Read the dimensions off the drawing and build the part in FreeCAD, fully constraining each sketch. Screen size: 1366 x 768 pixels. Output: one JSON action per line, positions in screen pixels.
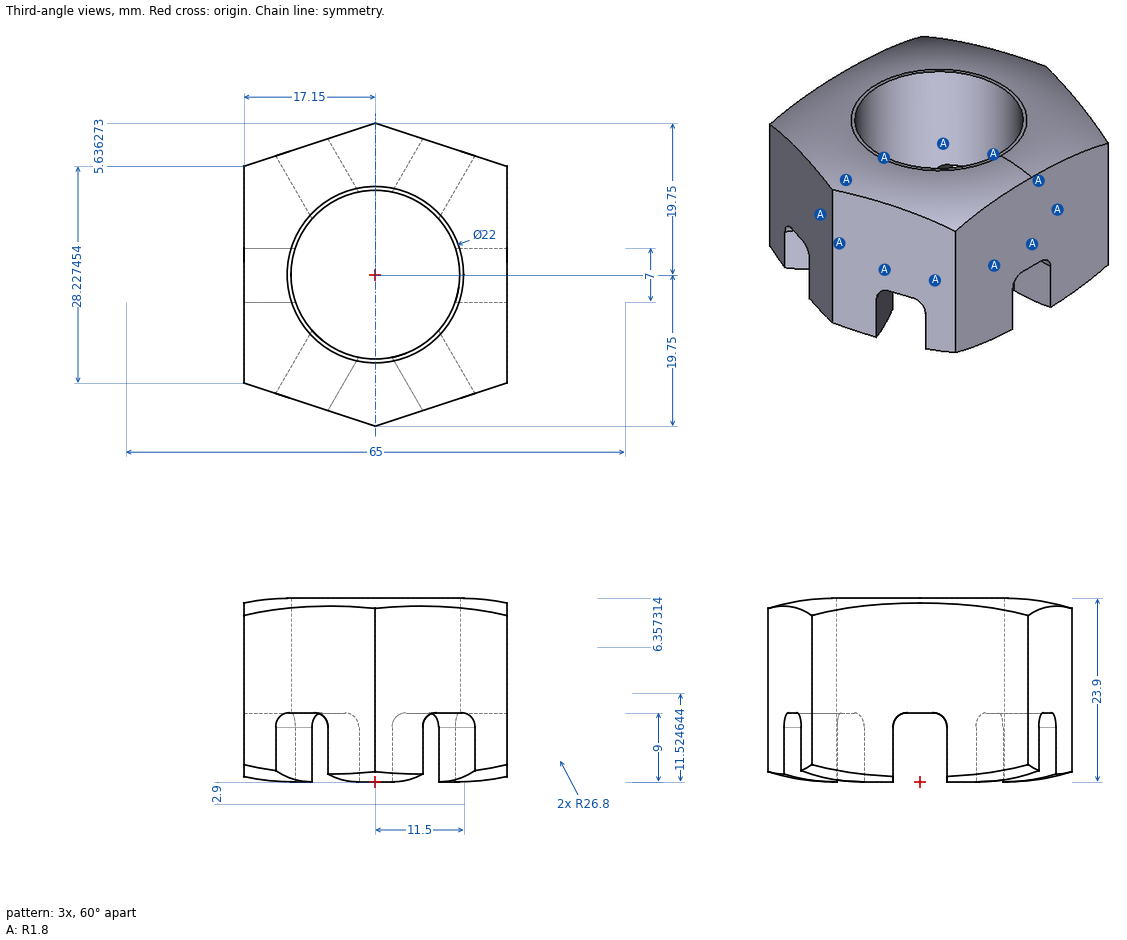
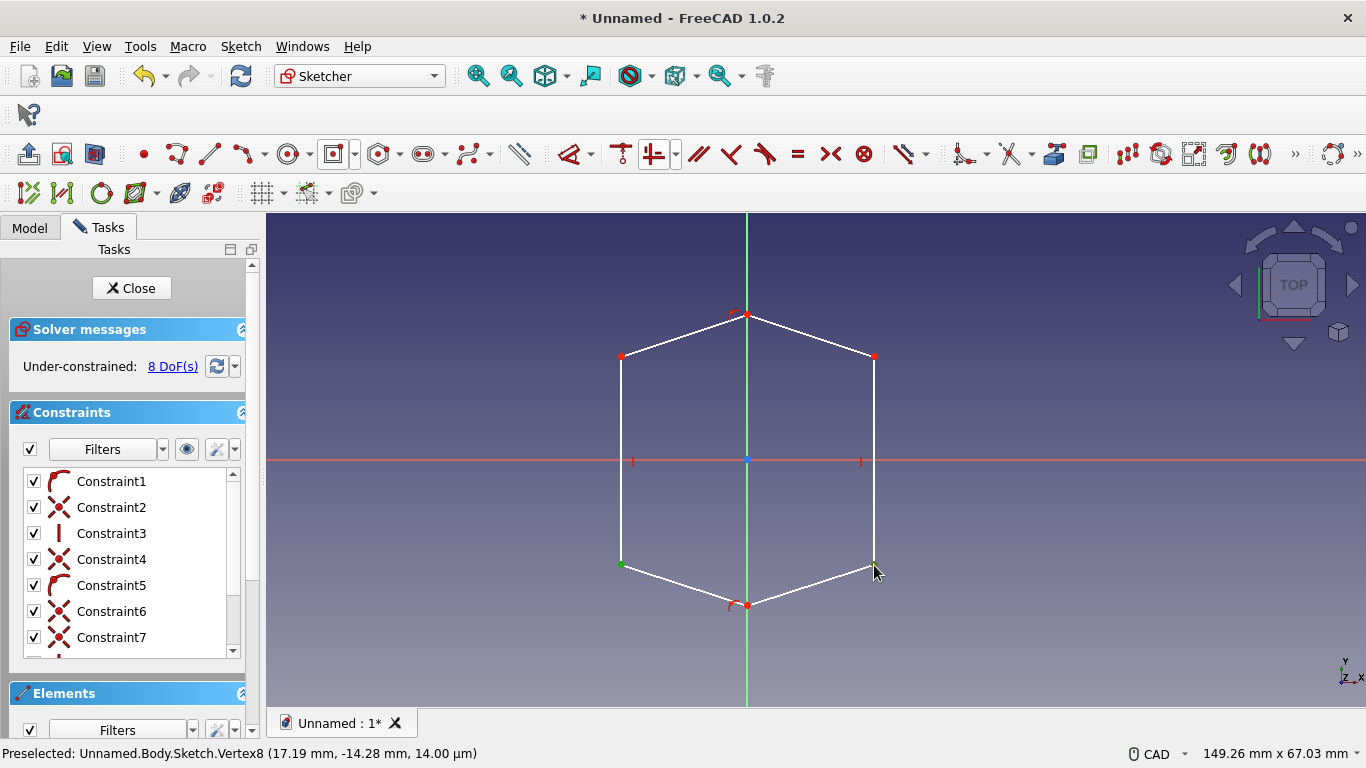
{"action": "left_click", "coordinate": [747, 648]}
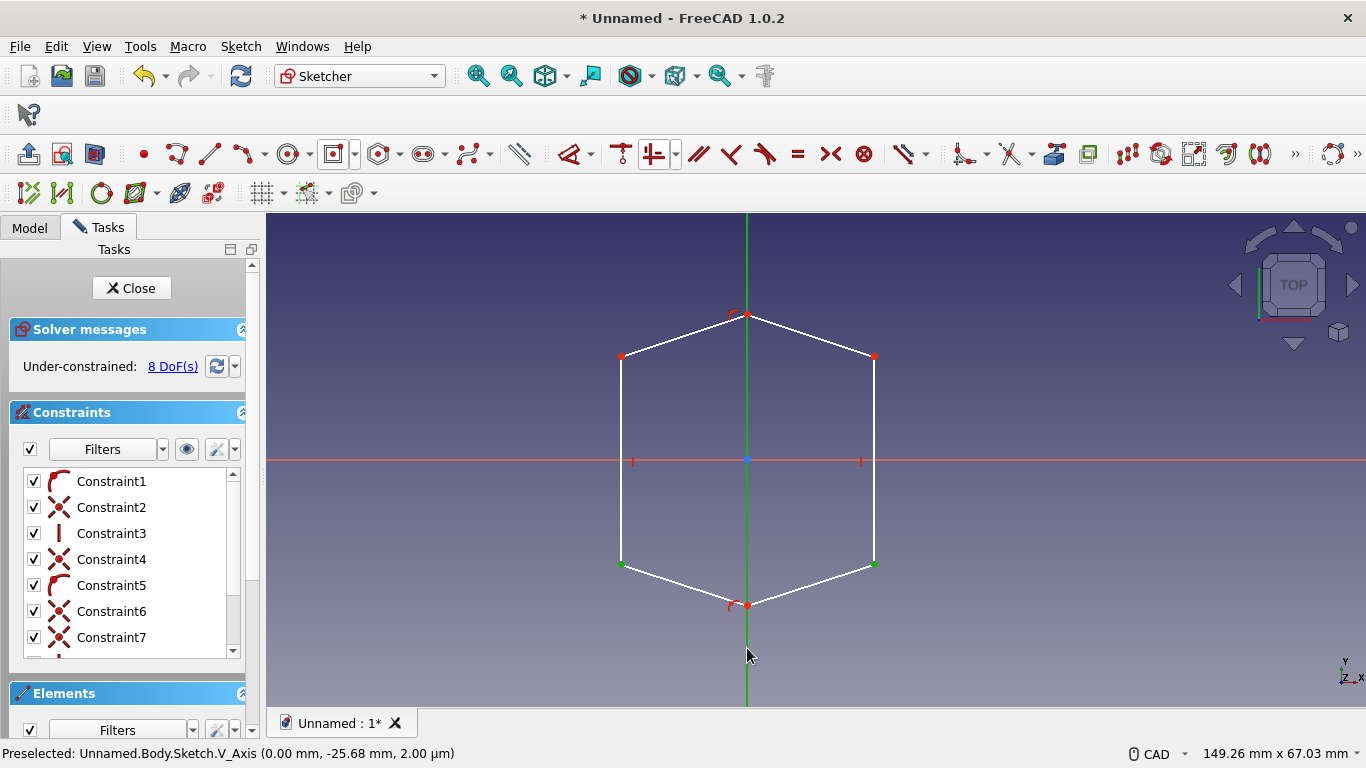
{"action": "left_click", "coordinate": [831, 154]}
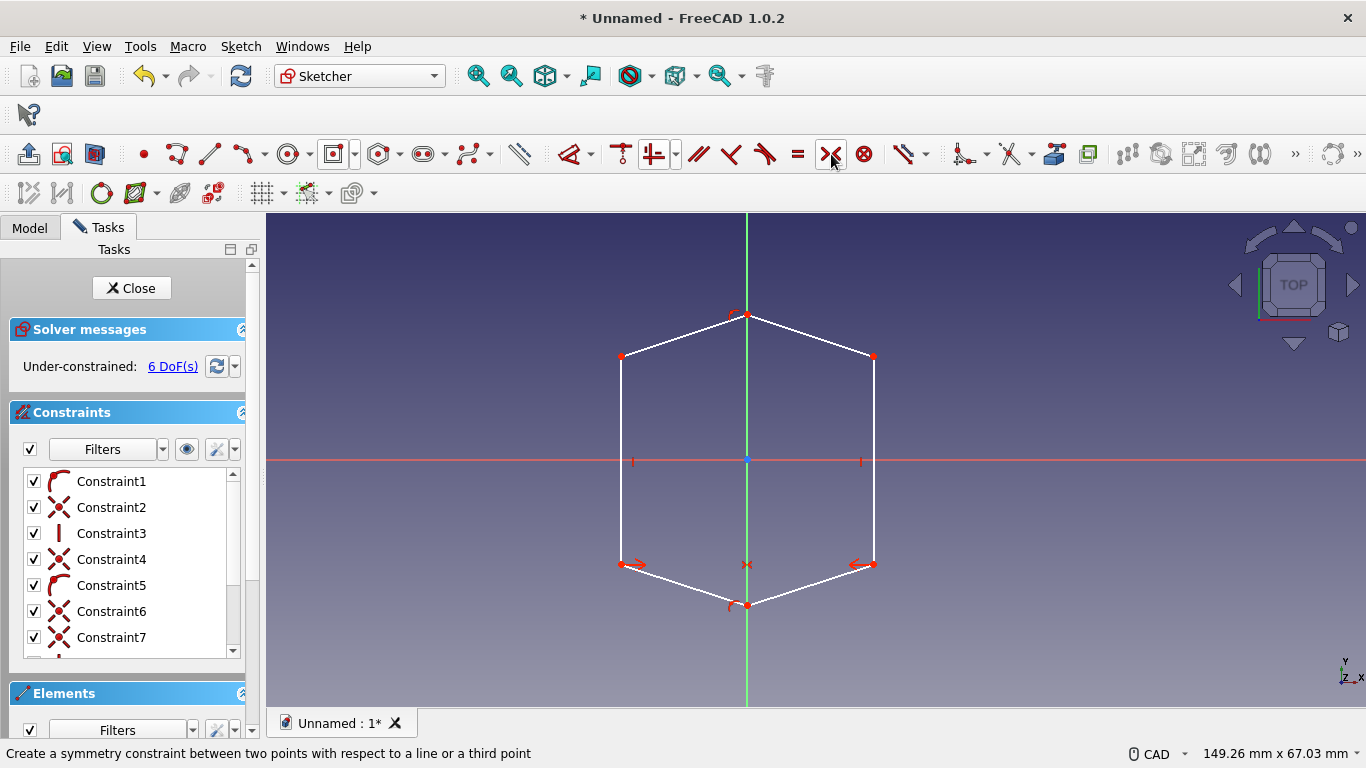
{"action": "left_click", "coordinate": [568, 154]}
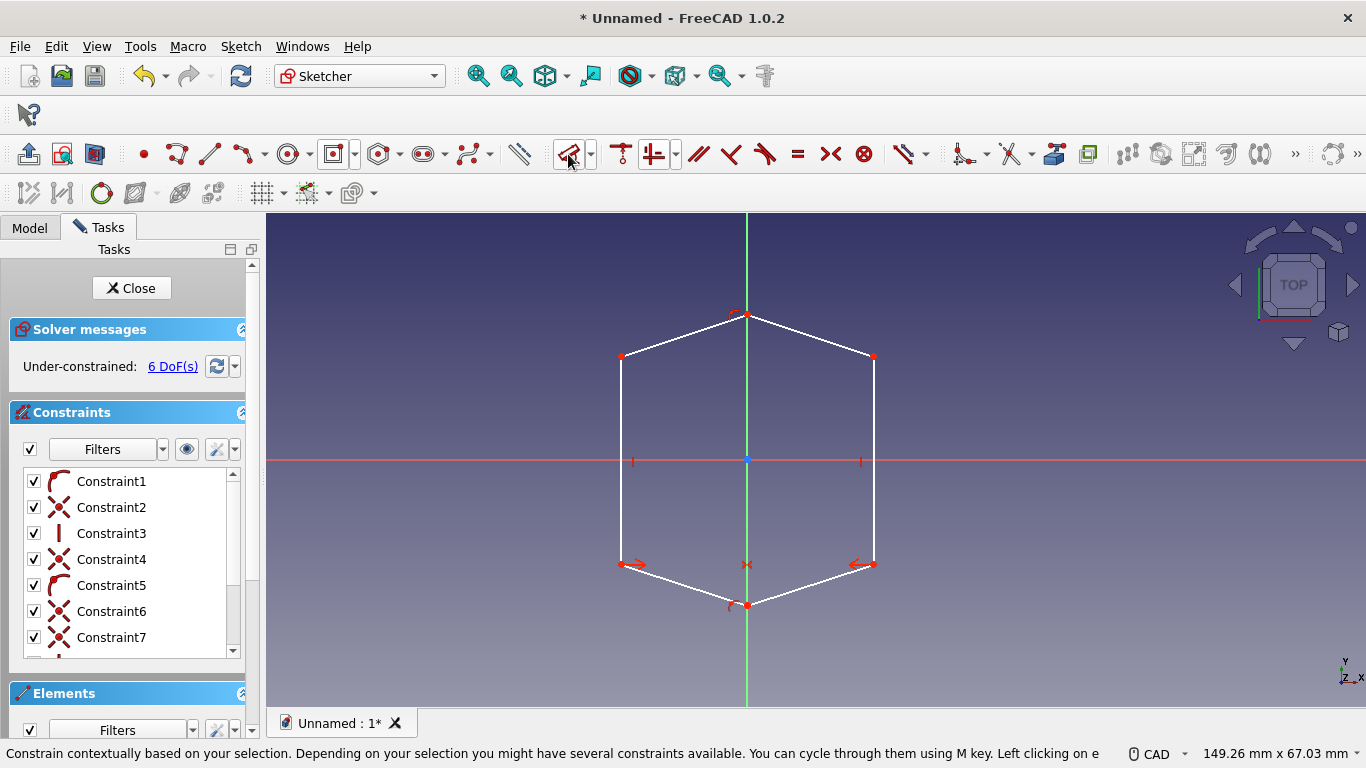
{"action": "left_click", "coordinate": [747, 315]}
{"action": "left_click", "coordinate": [781, 387]}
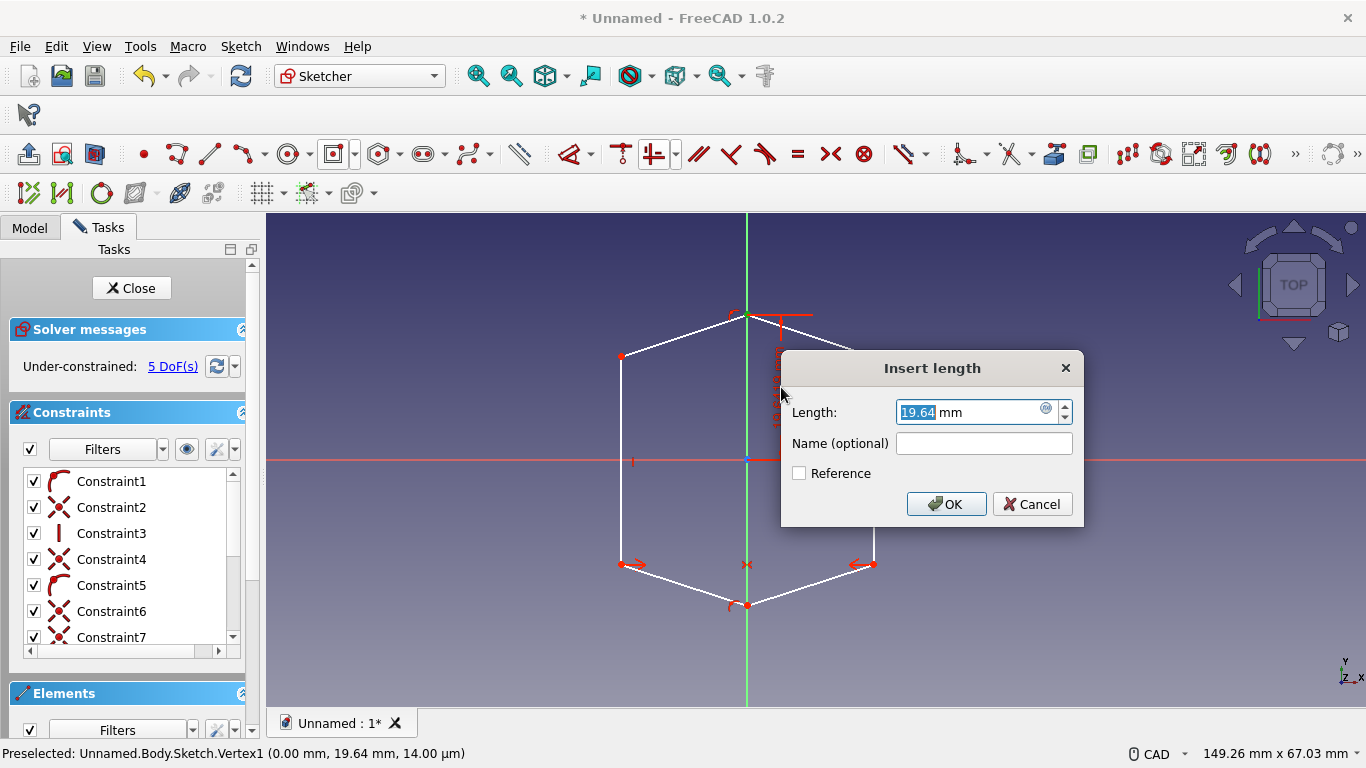
{"action": "type", "text": "19.75"}
{"action": "key", "text": "Return"}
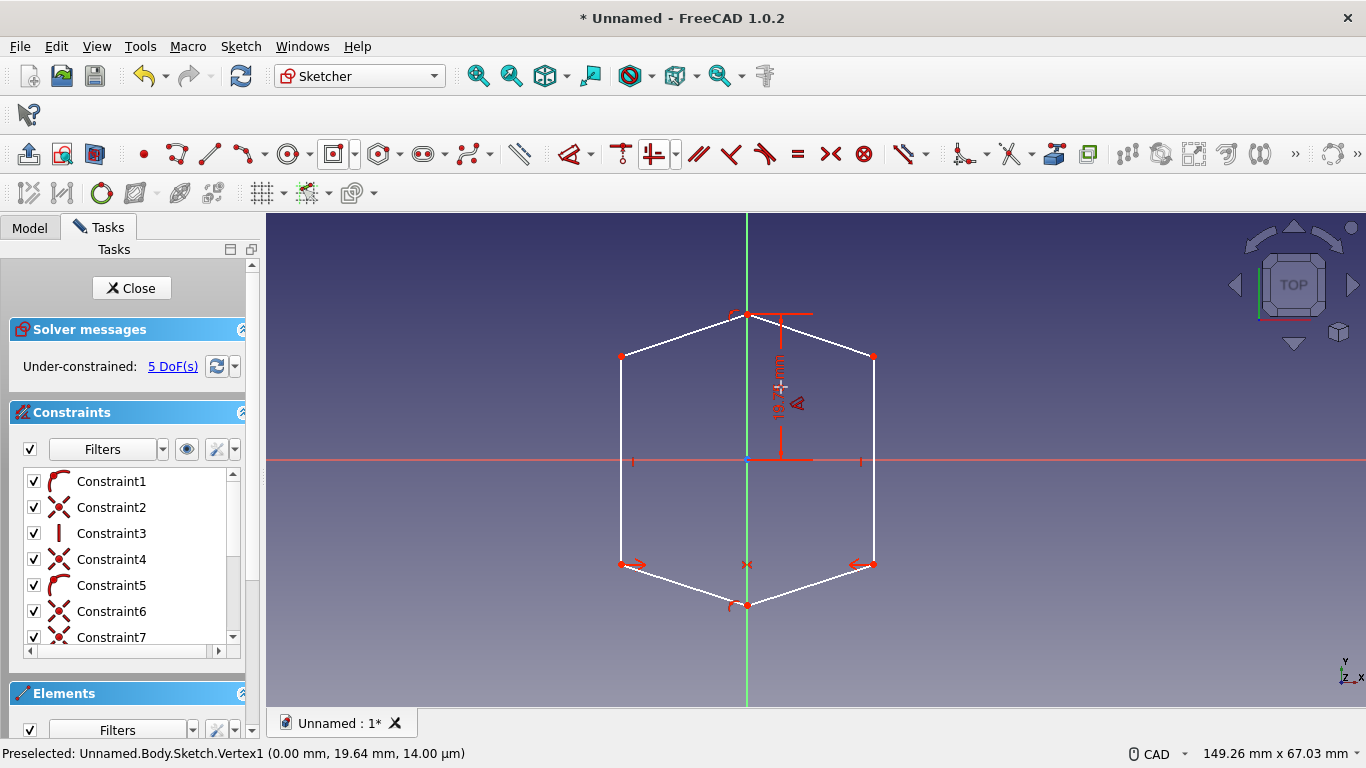
{"action": "left_click", "coordinate": [621, 357]}
{"action": "left_click", "coordinate": [655, 323]}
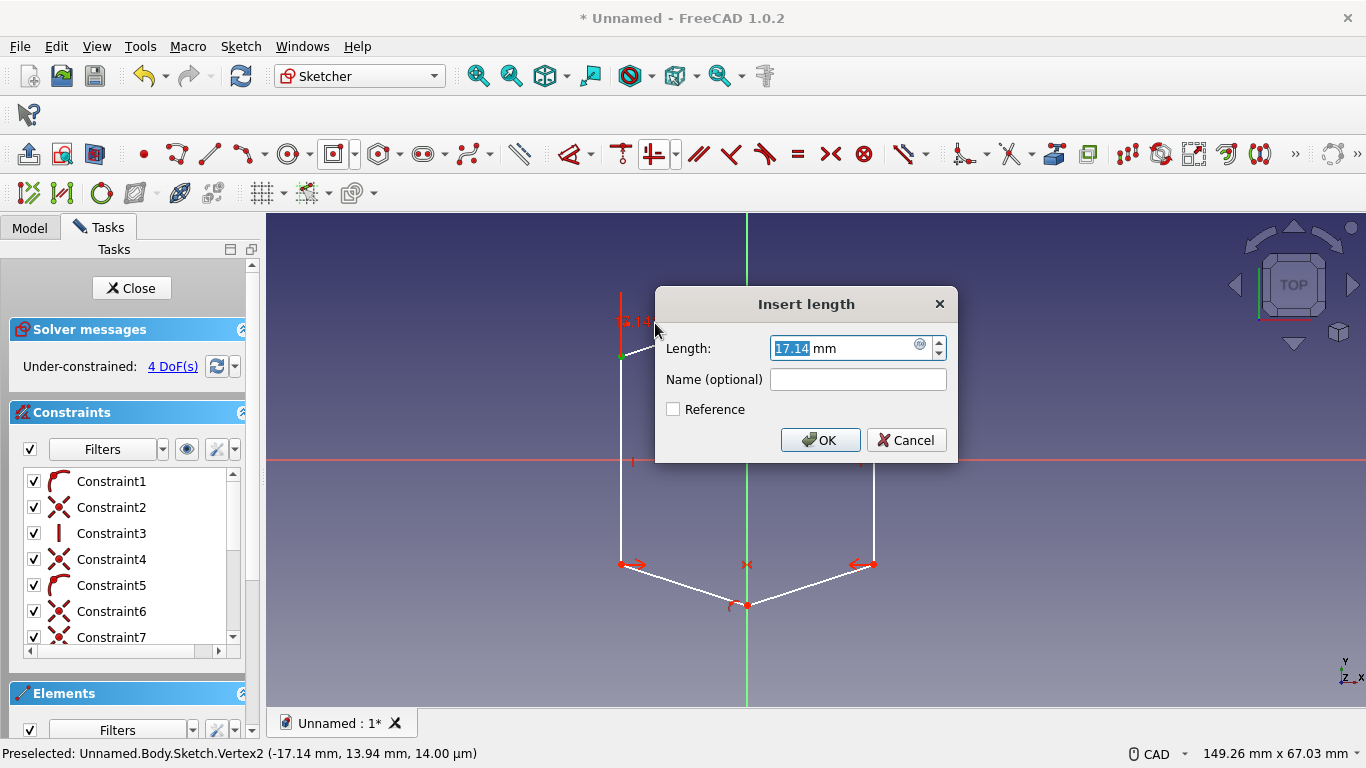
{"action": "type", "text": "17.15"}
{"action": "key", "text": "Return"}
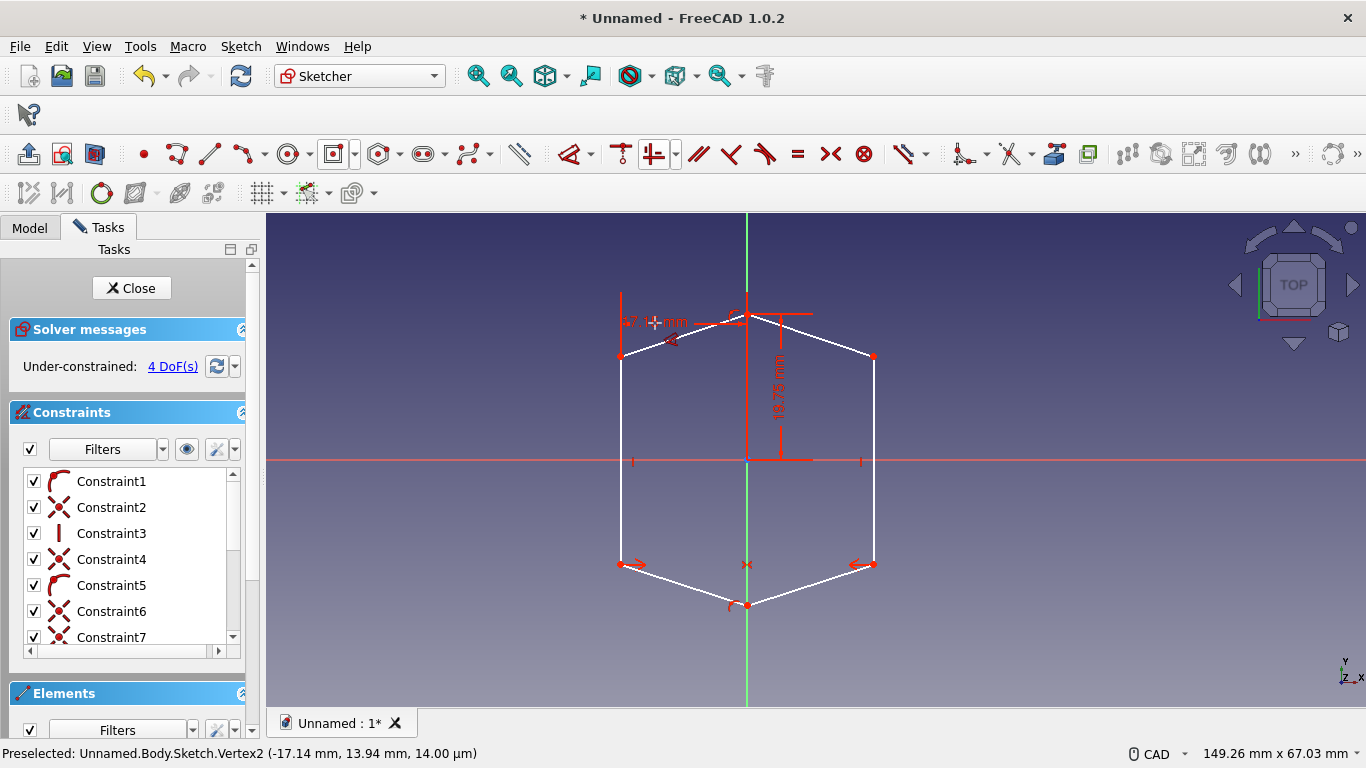
{"action": "left_click", "coordinate": [747, 606]}
{"action": "left_click", "coordinate": [781, 533]}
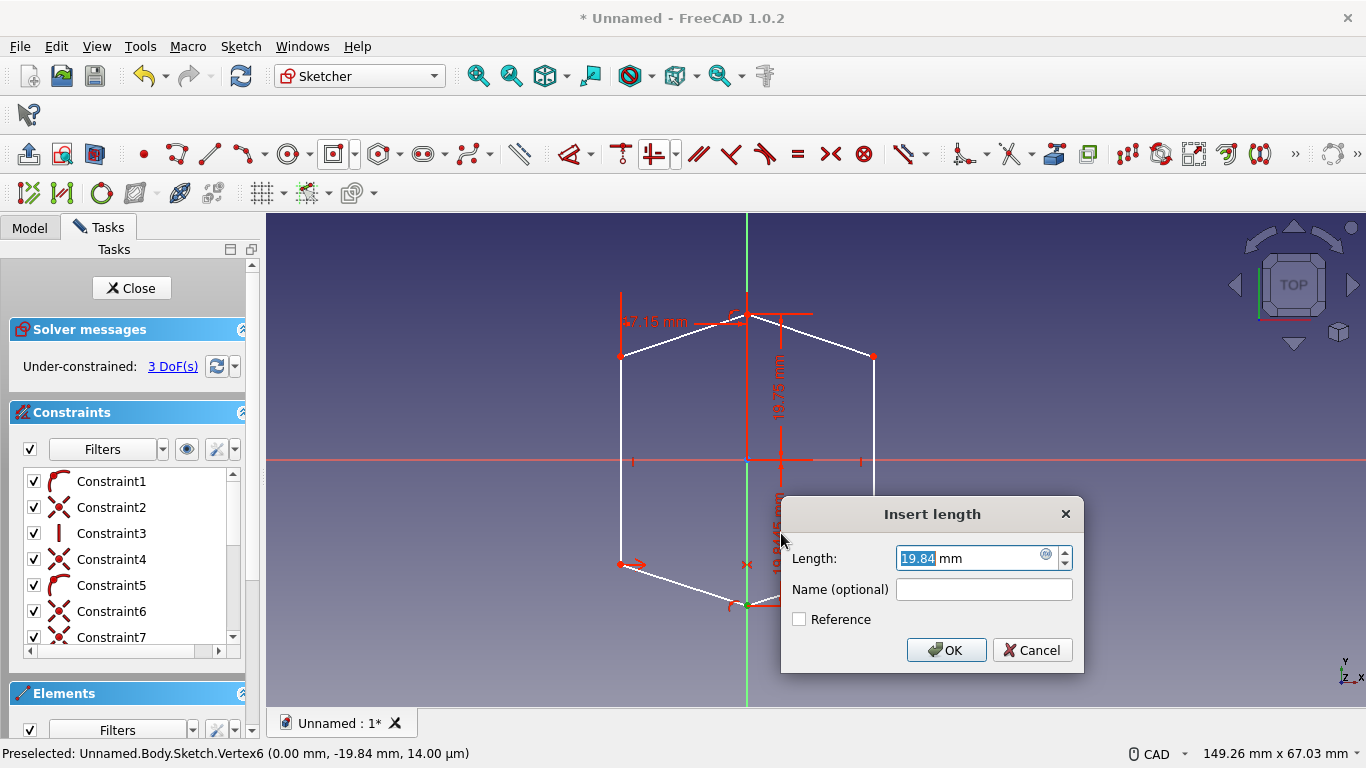
{"action": "type", "text": "19.75"}
{"action": "key", "text": "Return"}